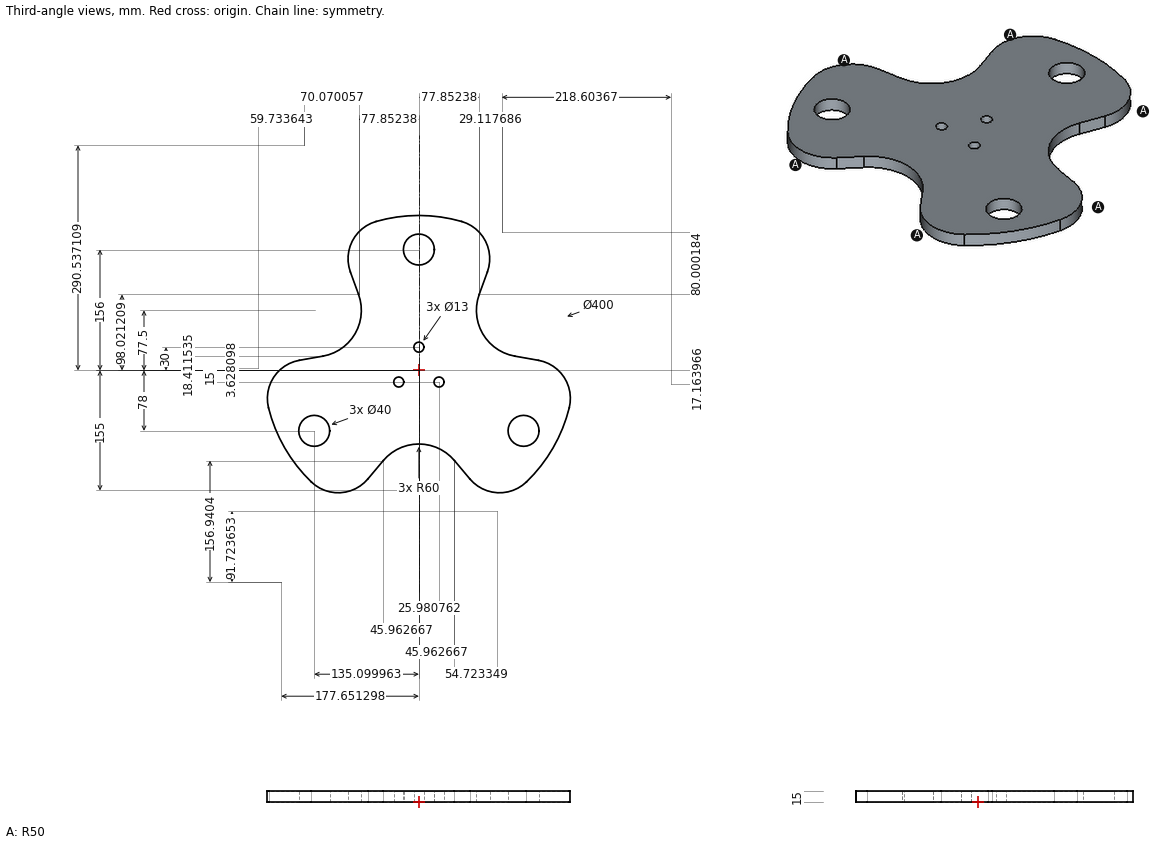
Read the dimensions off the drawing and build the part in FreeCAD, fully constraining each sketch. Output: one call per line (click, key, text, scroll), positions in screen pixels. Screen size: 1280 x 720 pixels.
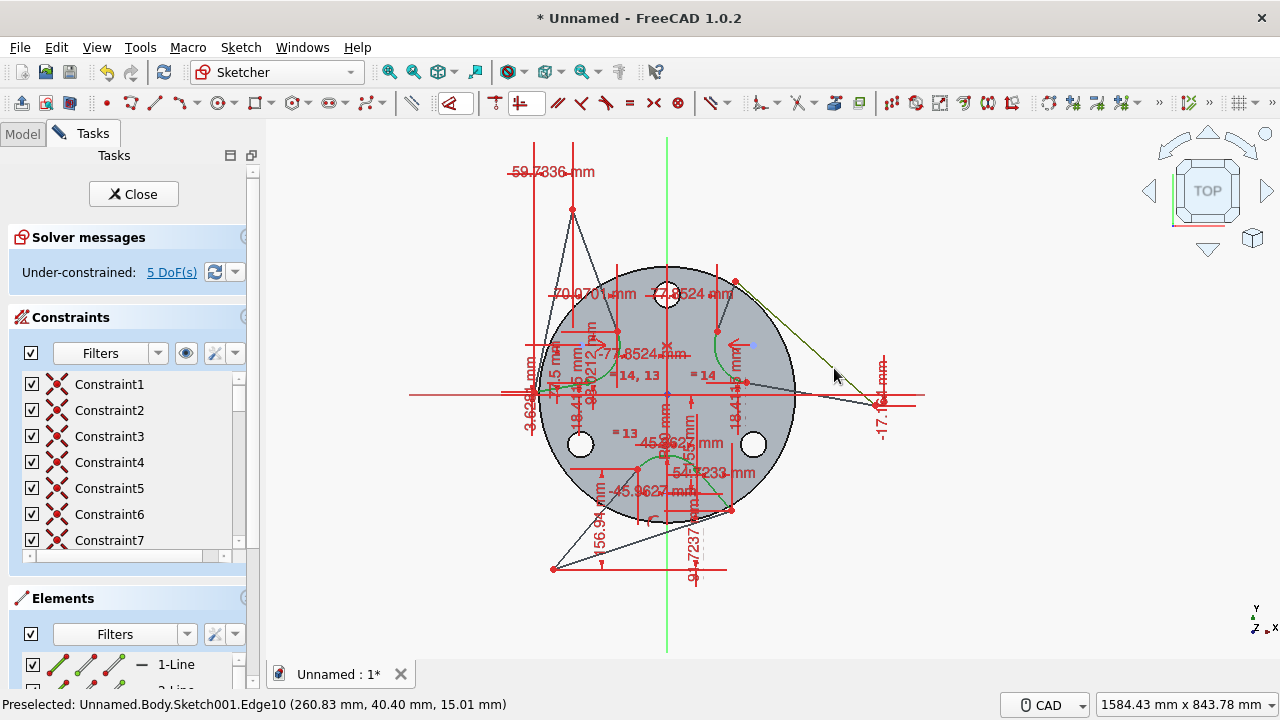
click(468, 104)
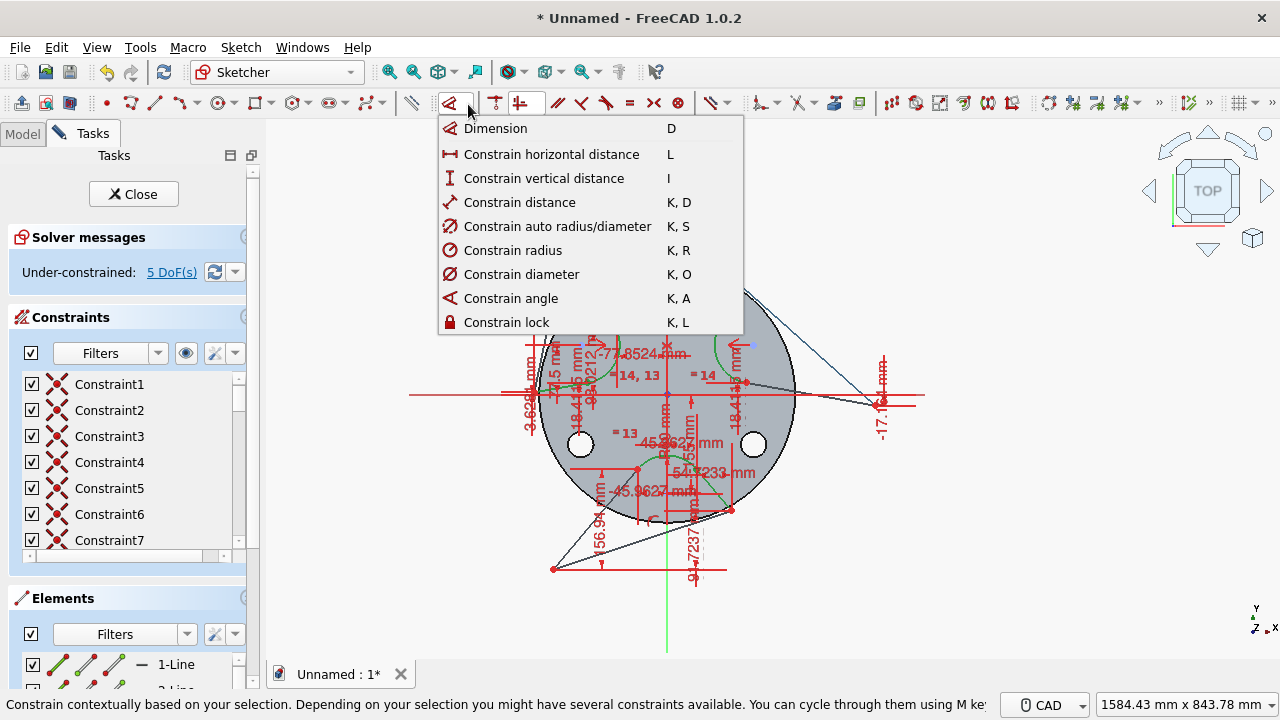
click(591, 154)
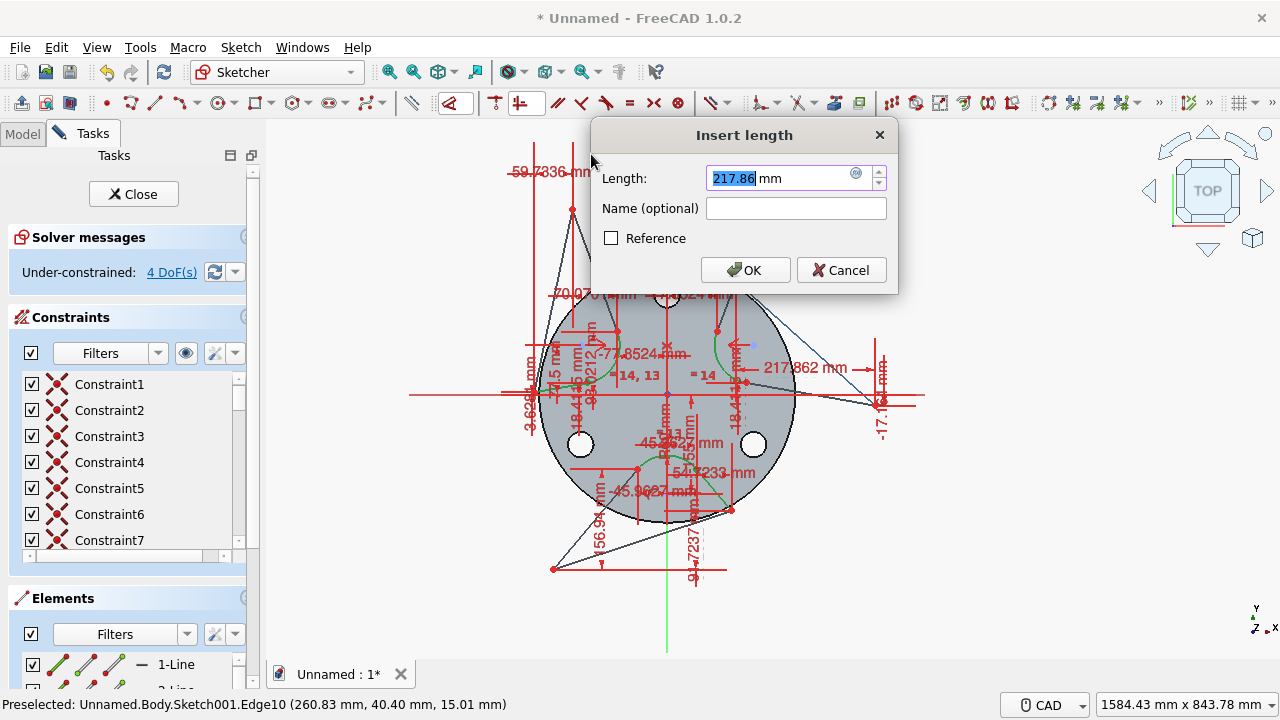
text(218.60367)
key(Return)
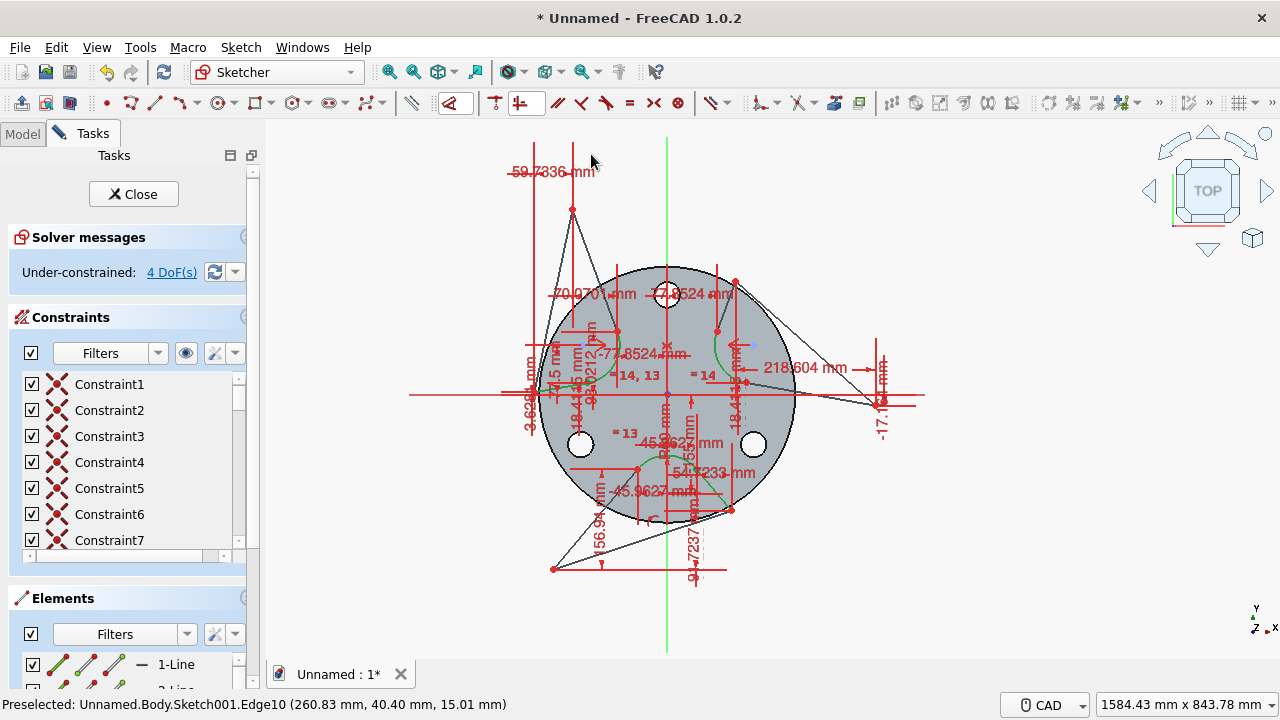
scroll(730, 296, up, 4)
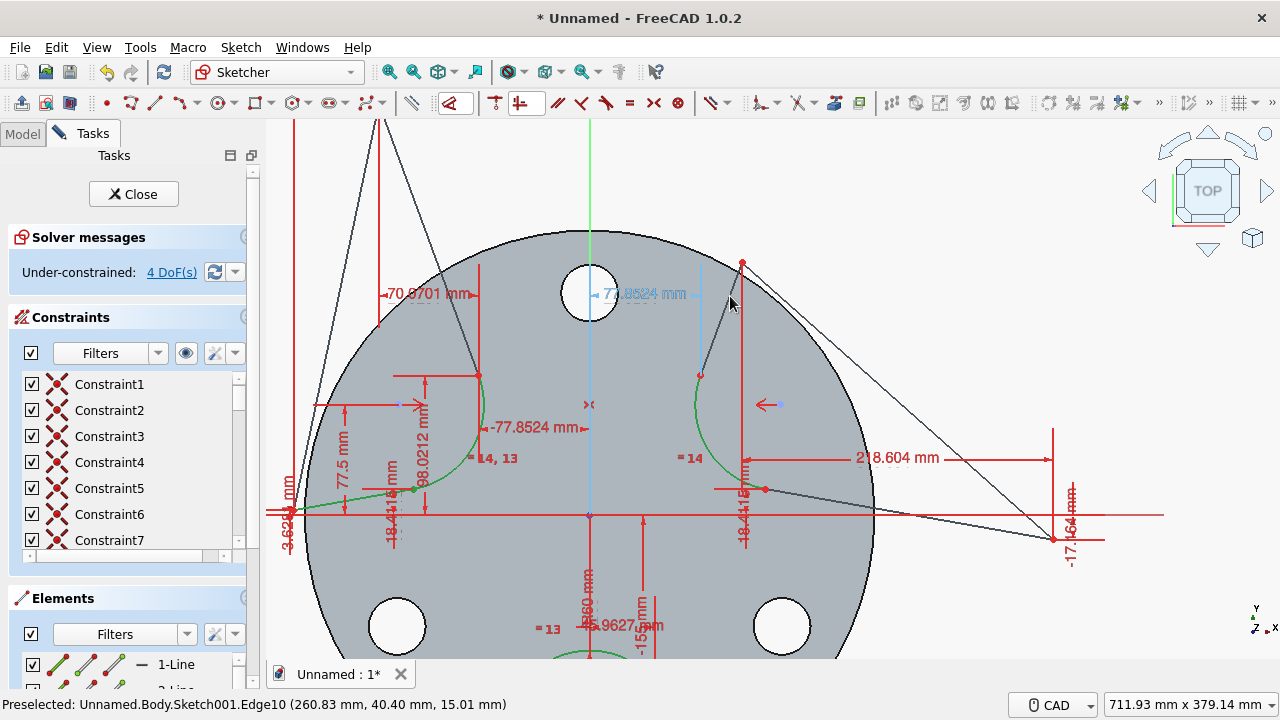
click(730, 297)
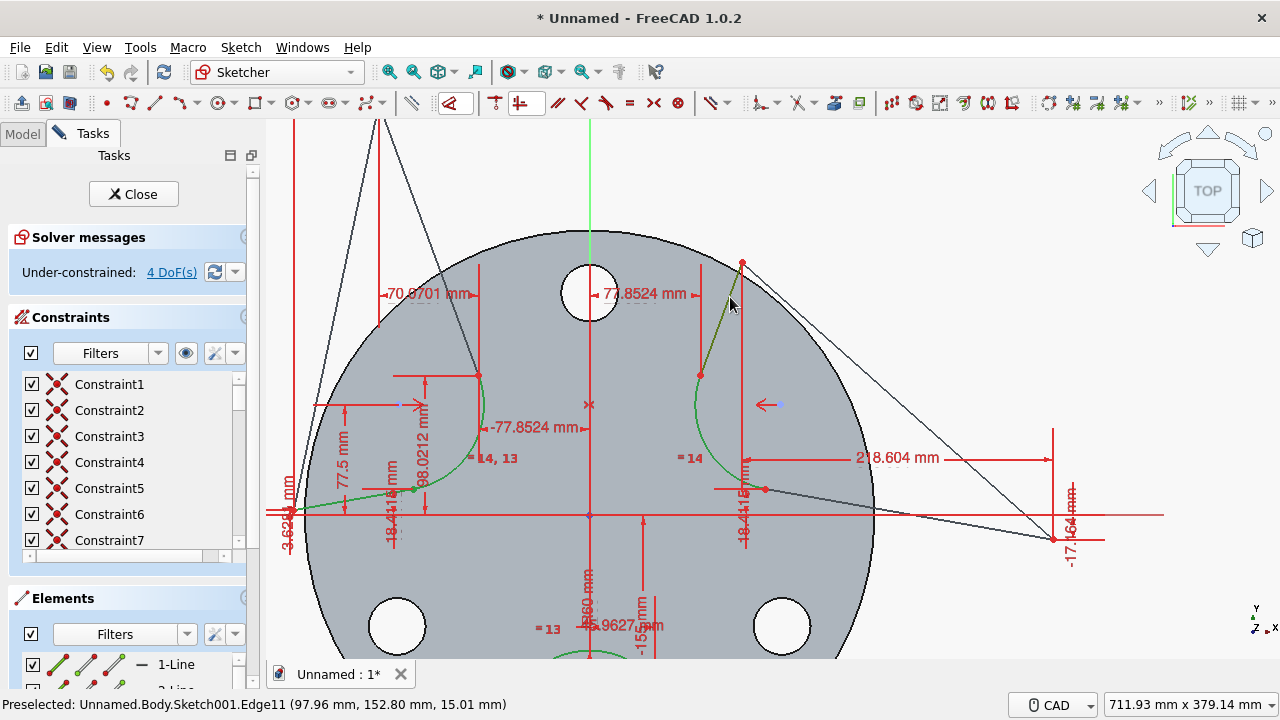
key(l)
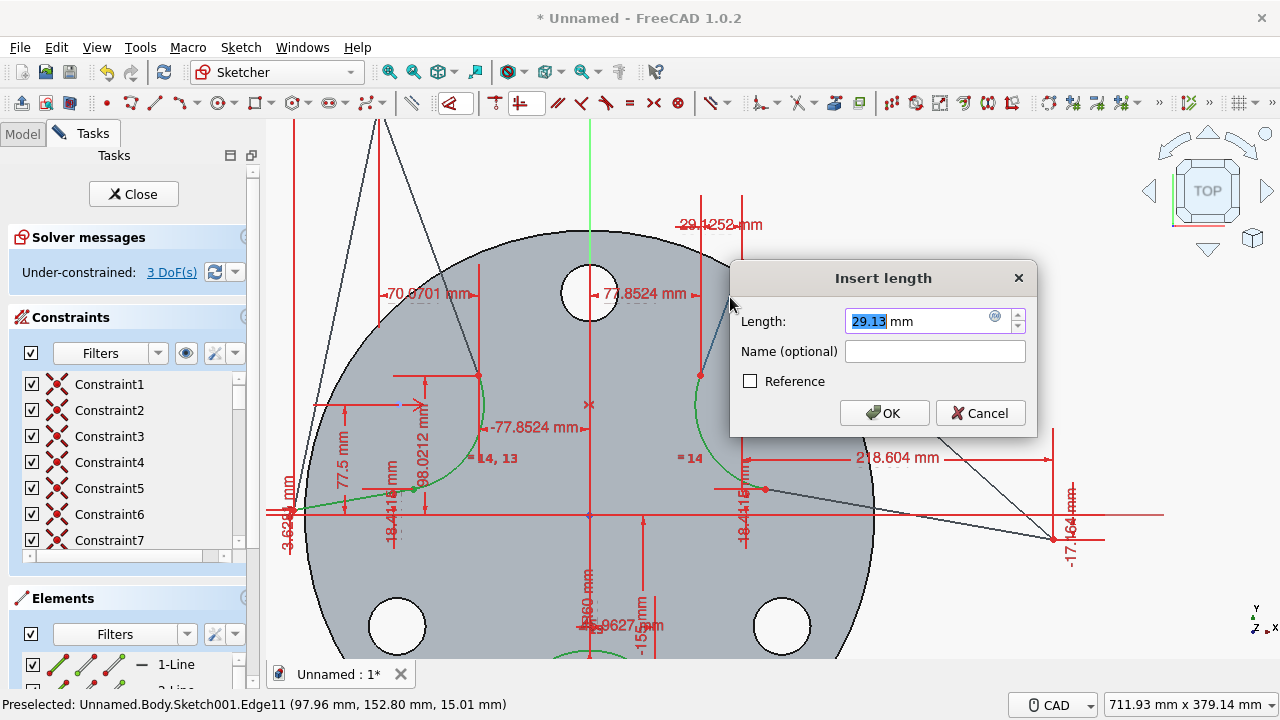
text(29.117686)
key(Return)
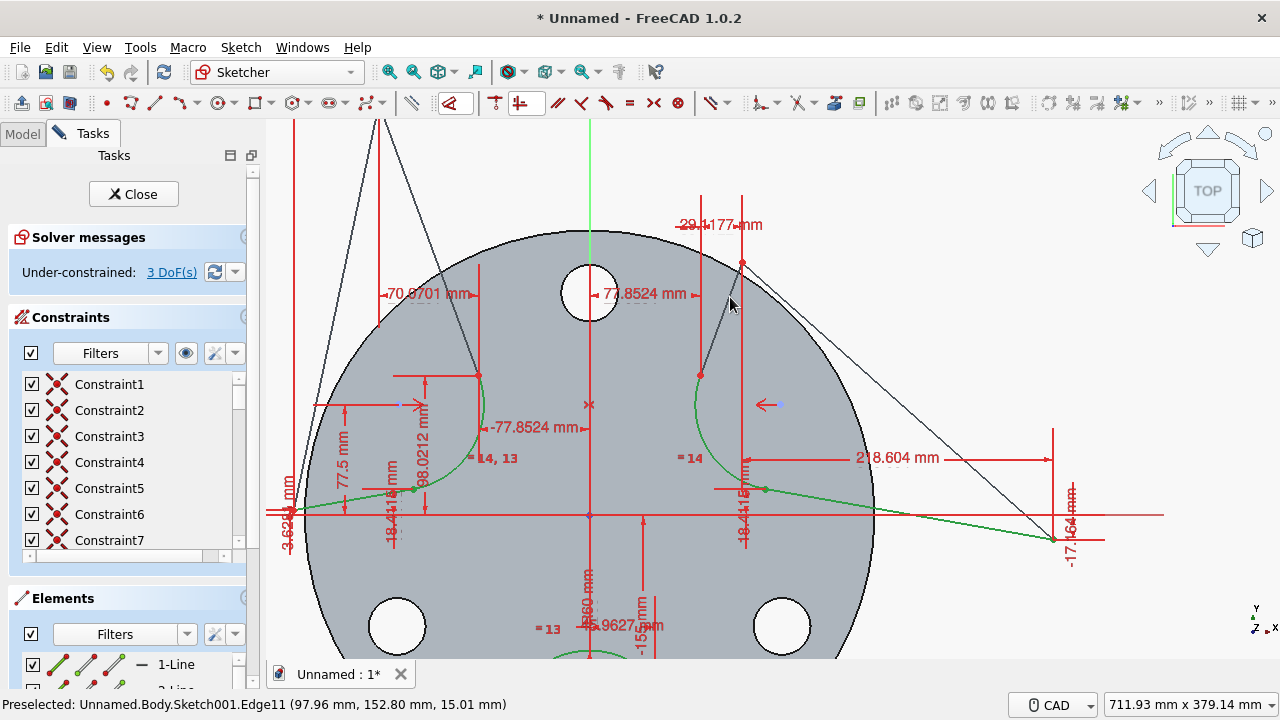
click(730, 297)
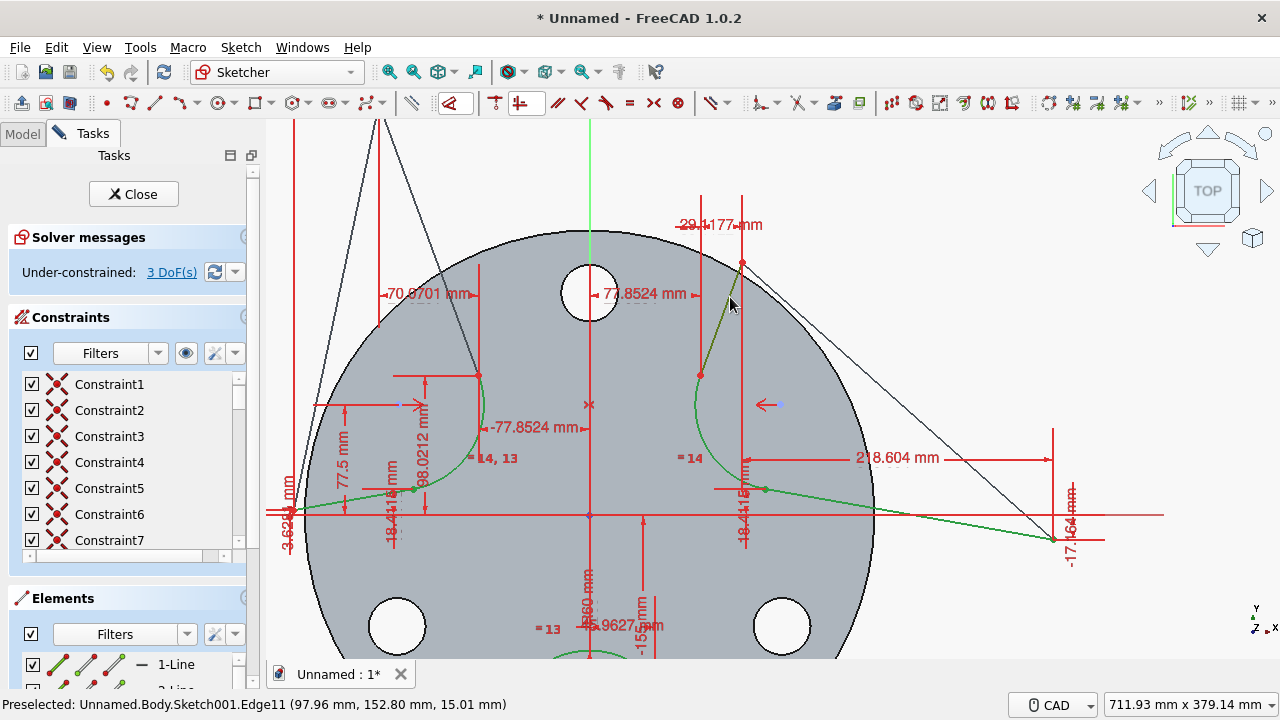
key(i)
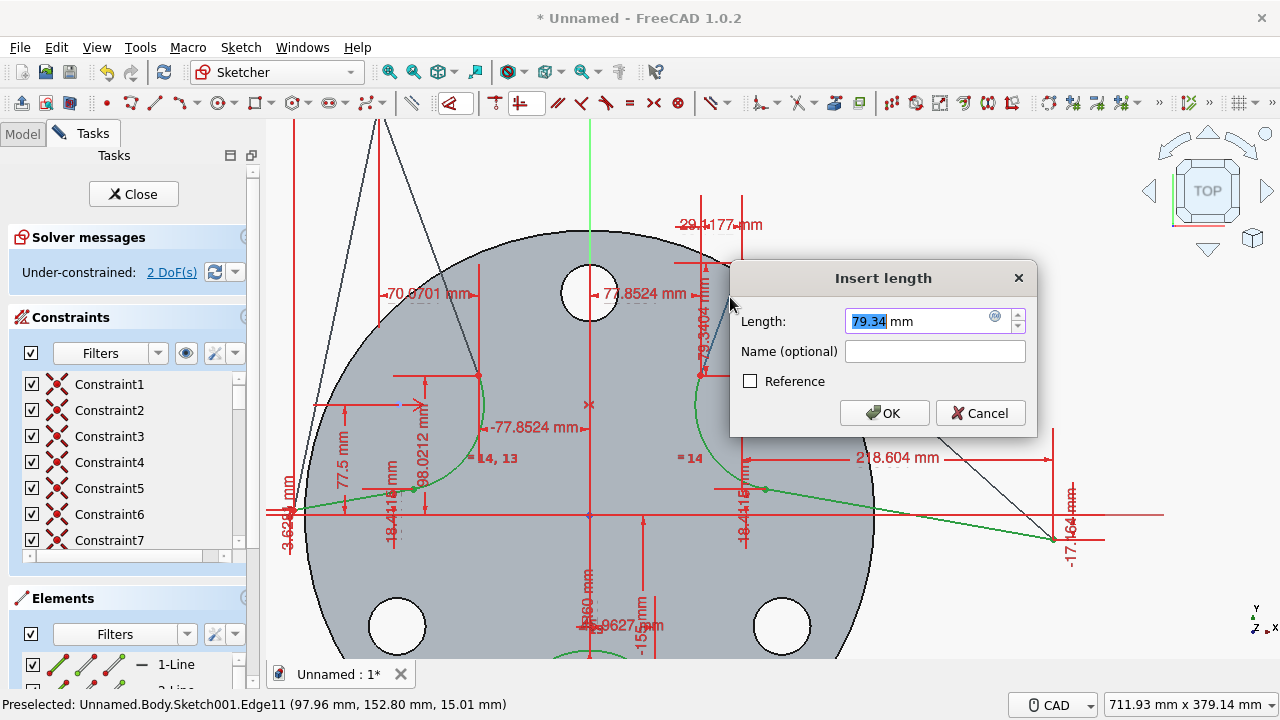
text(80.000184)
key(Return)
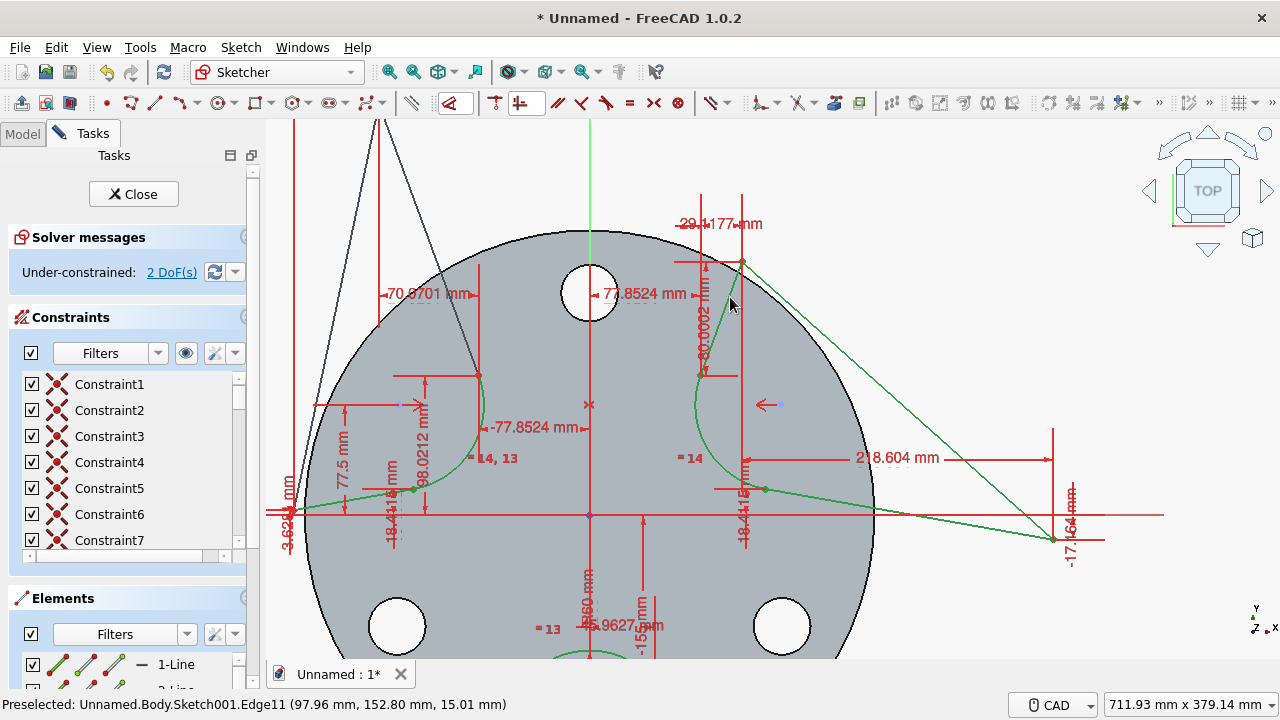
scroll(730, 296, down, 4)